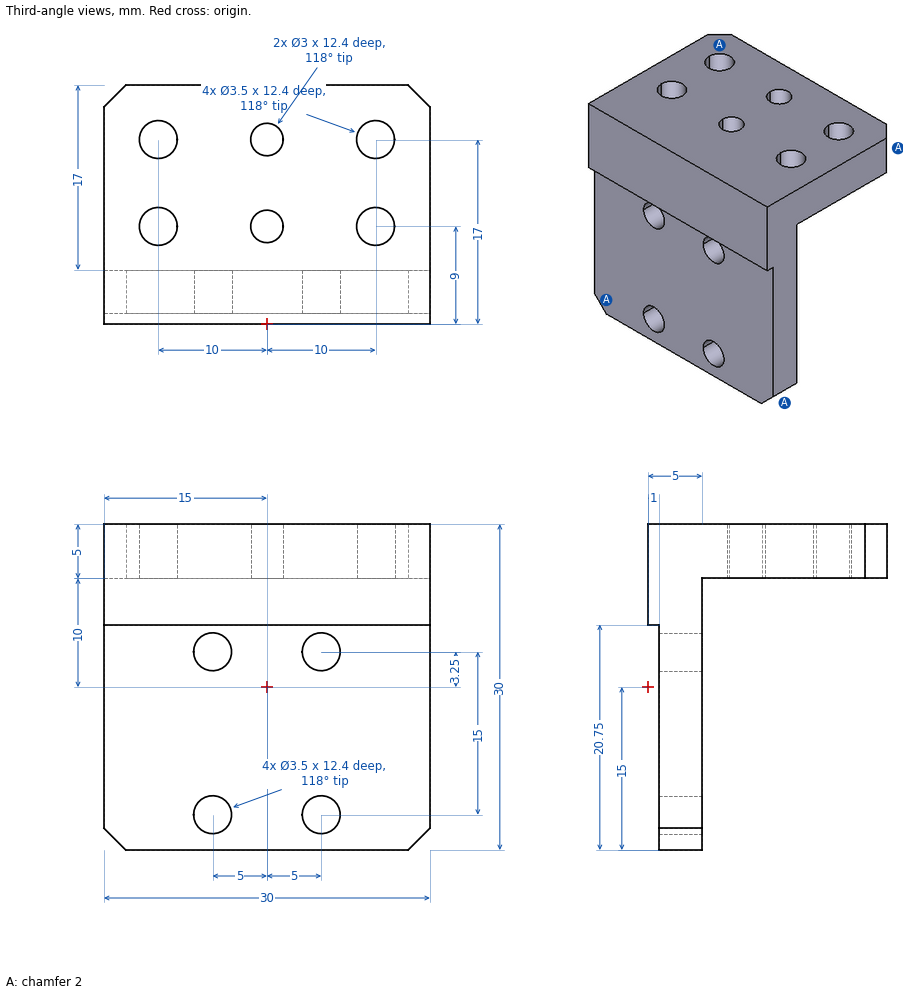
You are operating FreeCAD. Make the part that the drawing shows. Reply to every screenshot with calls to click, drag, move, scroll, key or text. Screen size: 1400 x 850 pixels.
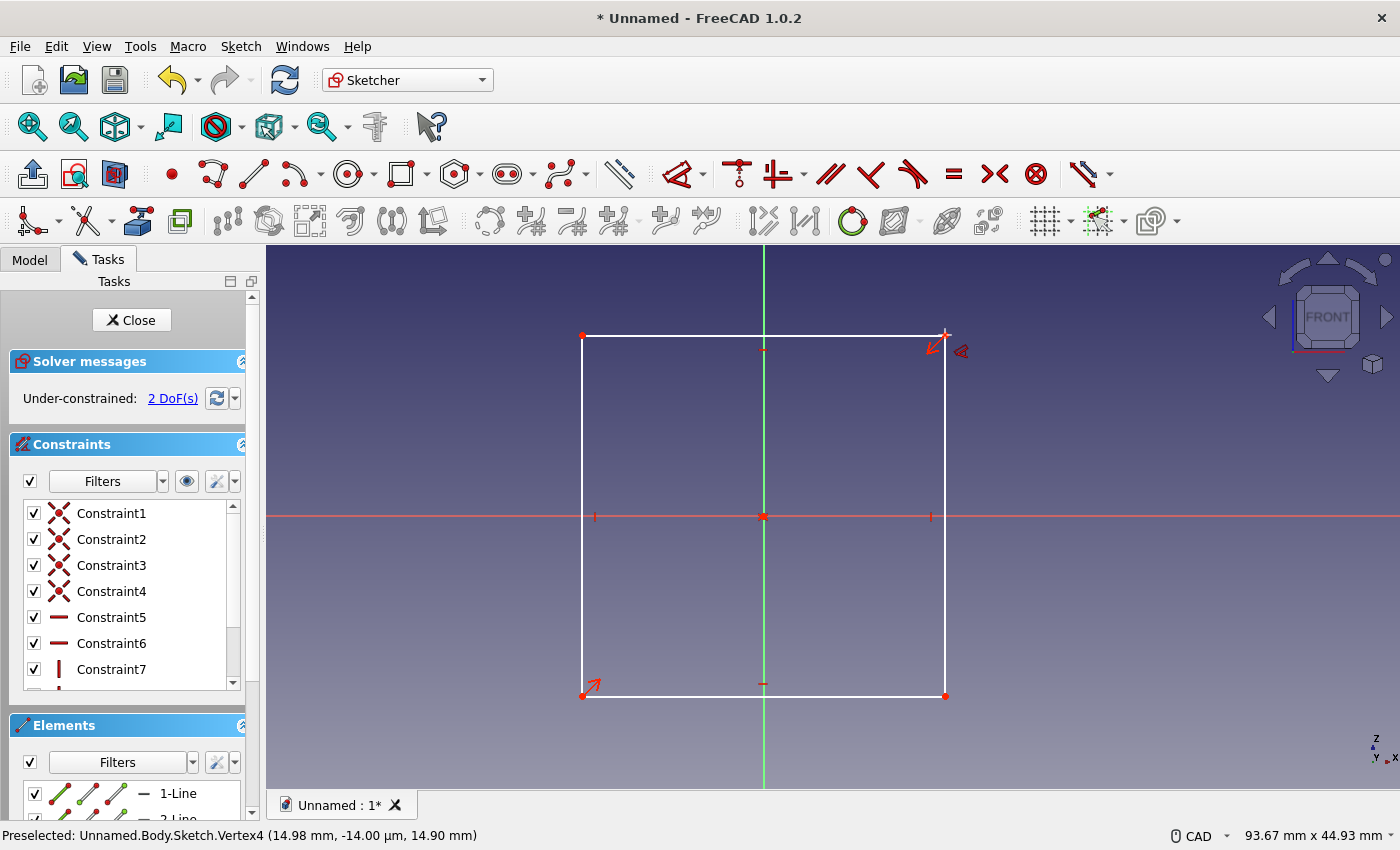
click(691, 697)
click(680, 731)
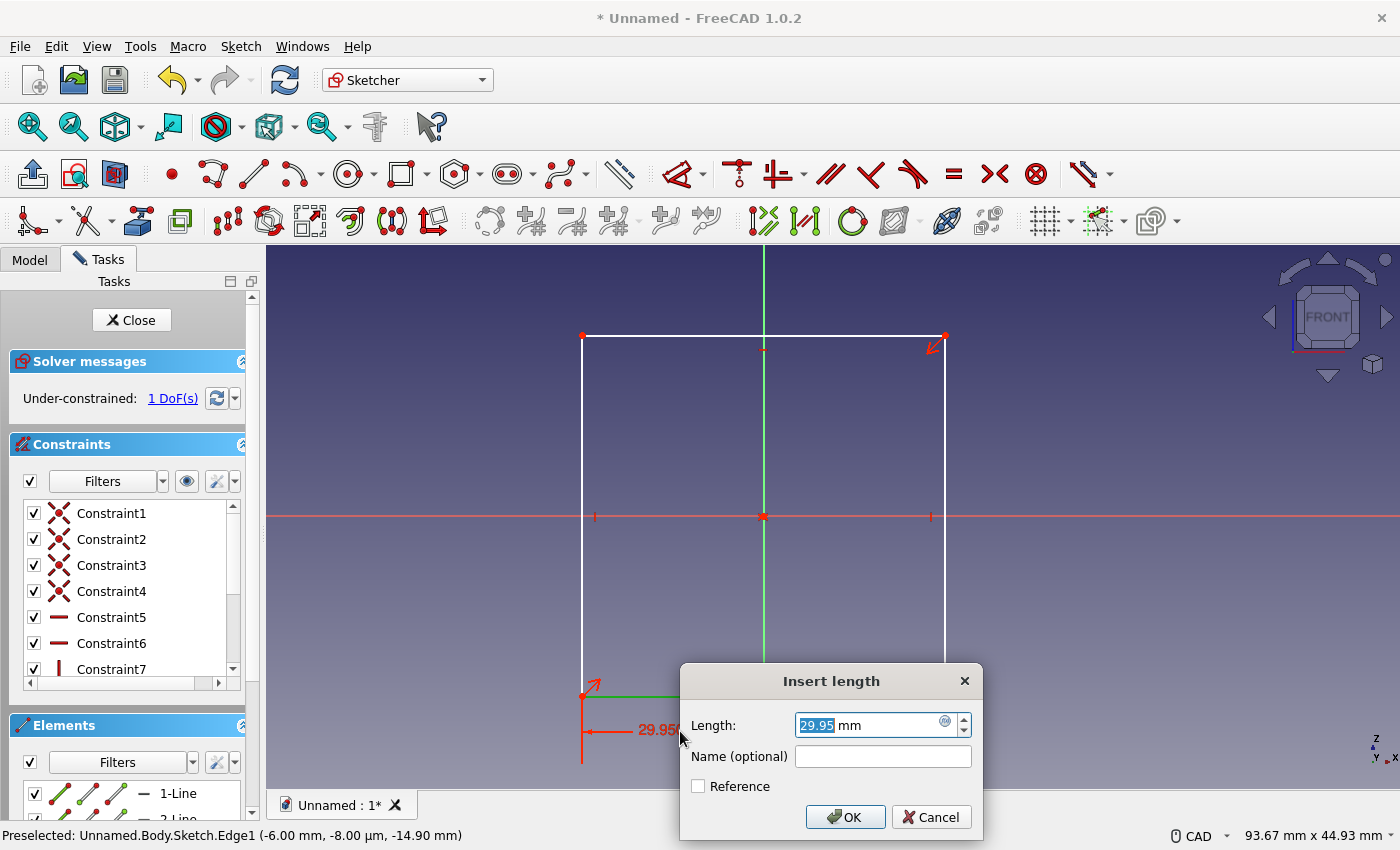
text(30)
key(Return)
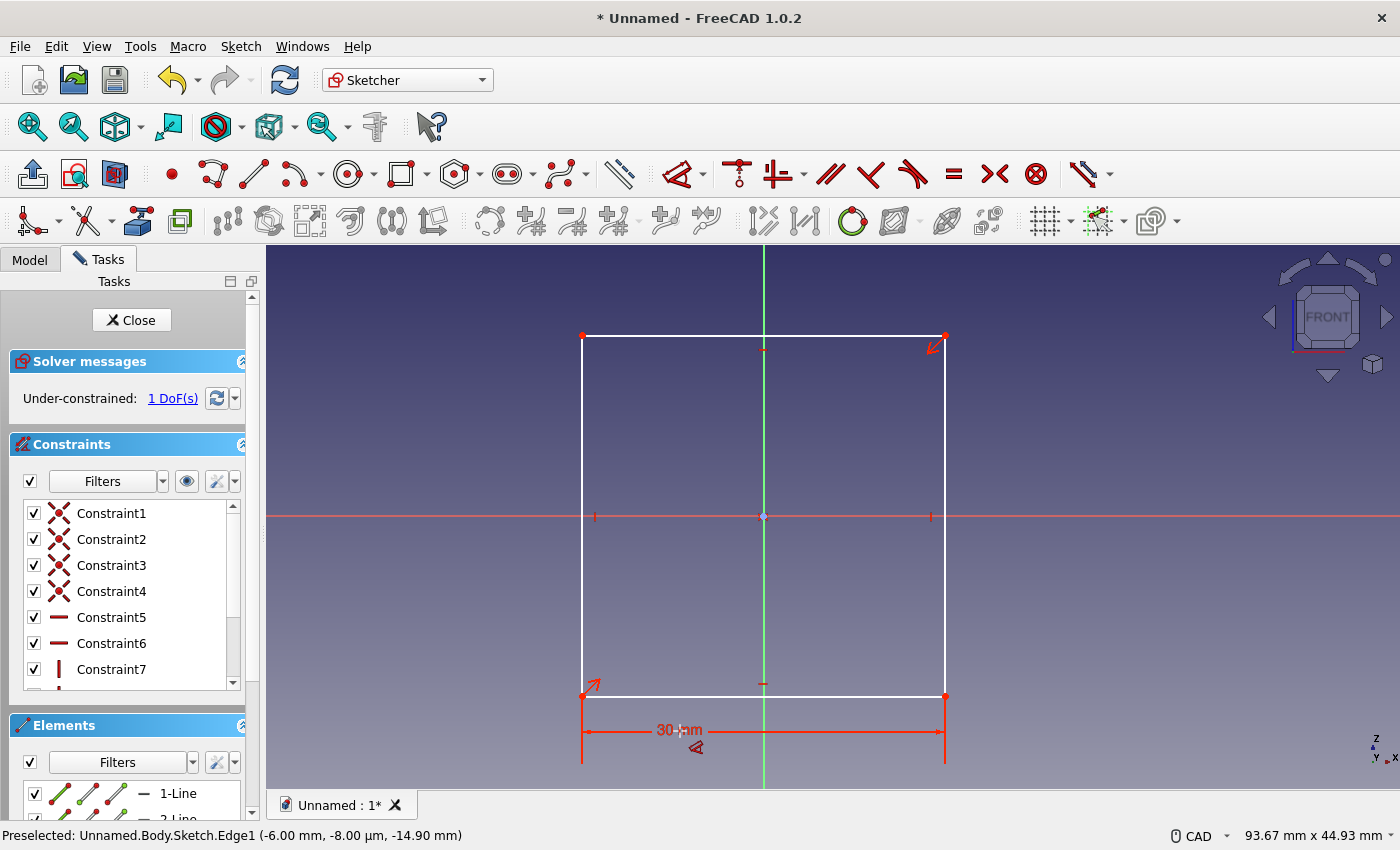
click(945, 589)
click(979, 433)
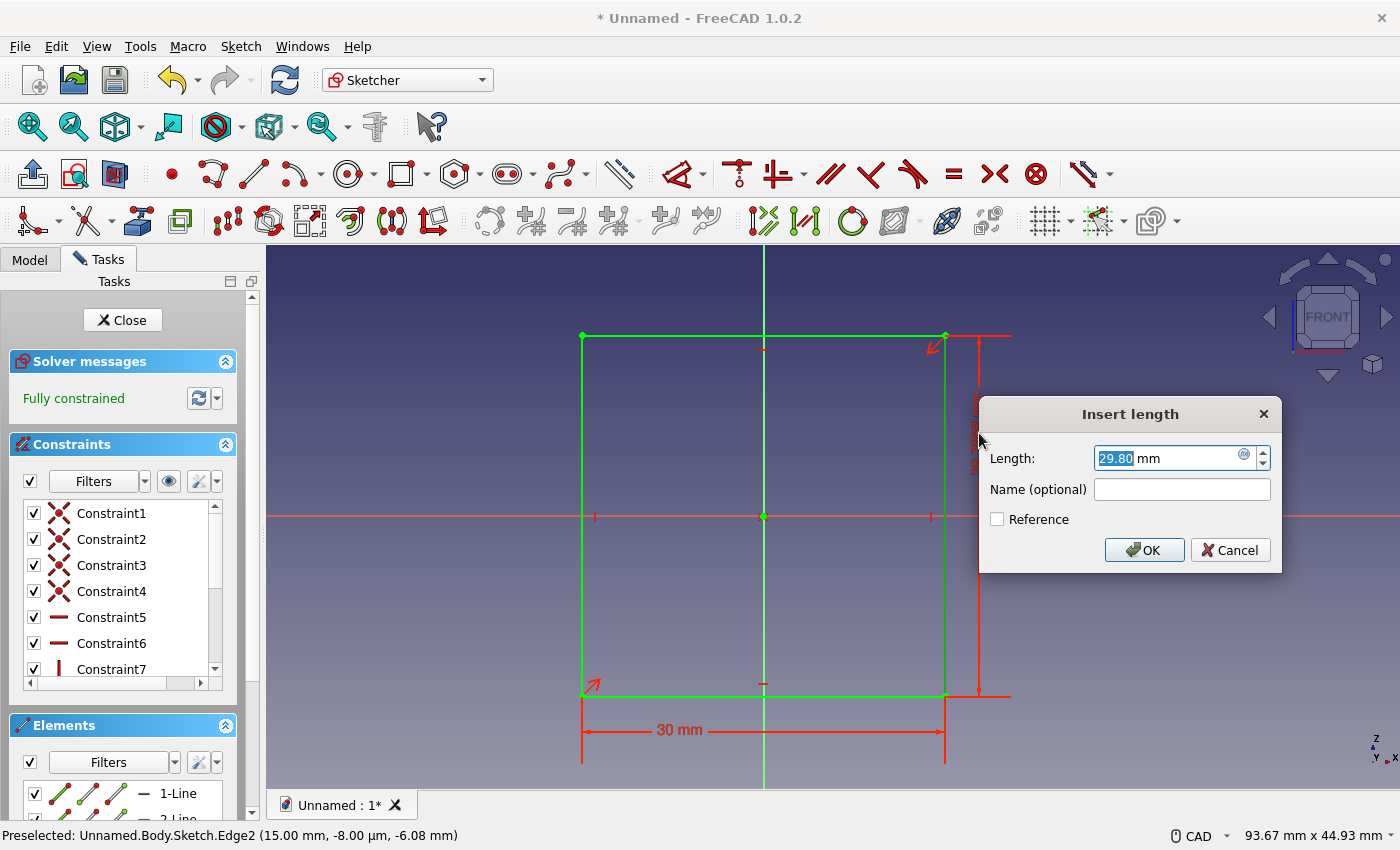
text(30)
key(Return)
key(Escape)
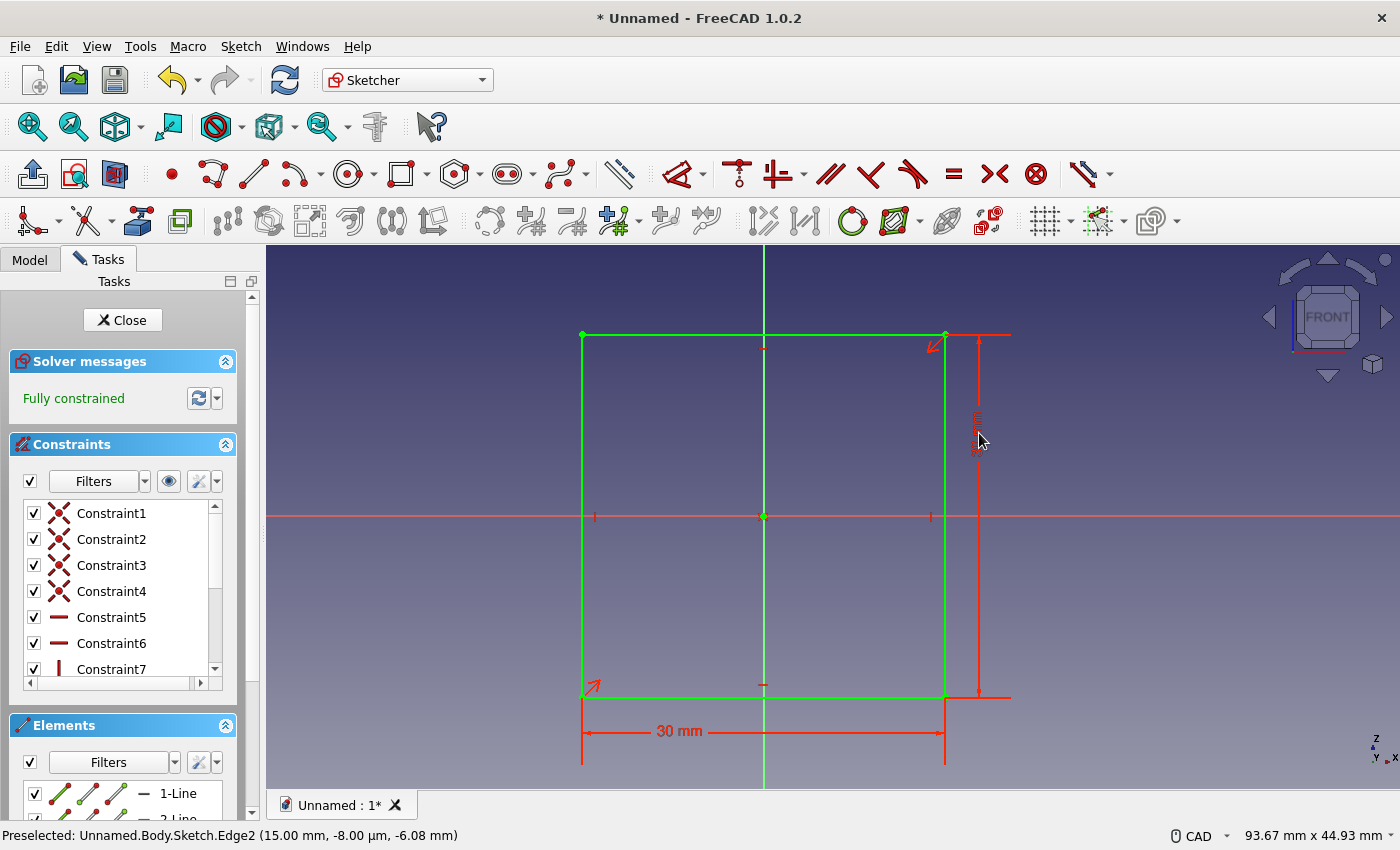
click(123, 320)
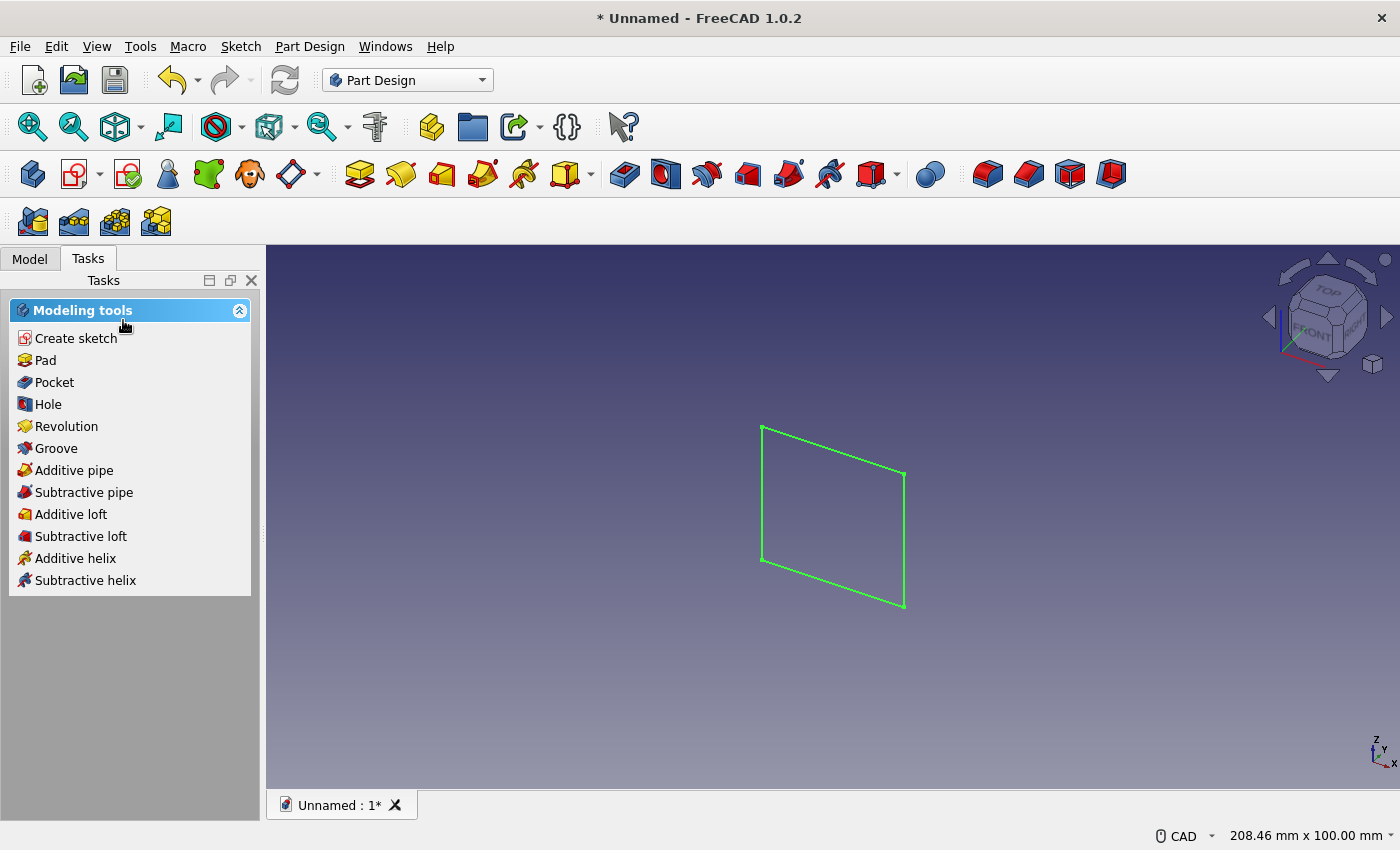
click(360, 174)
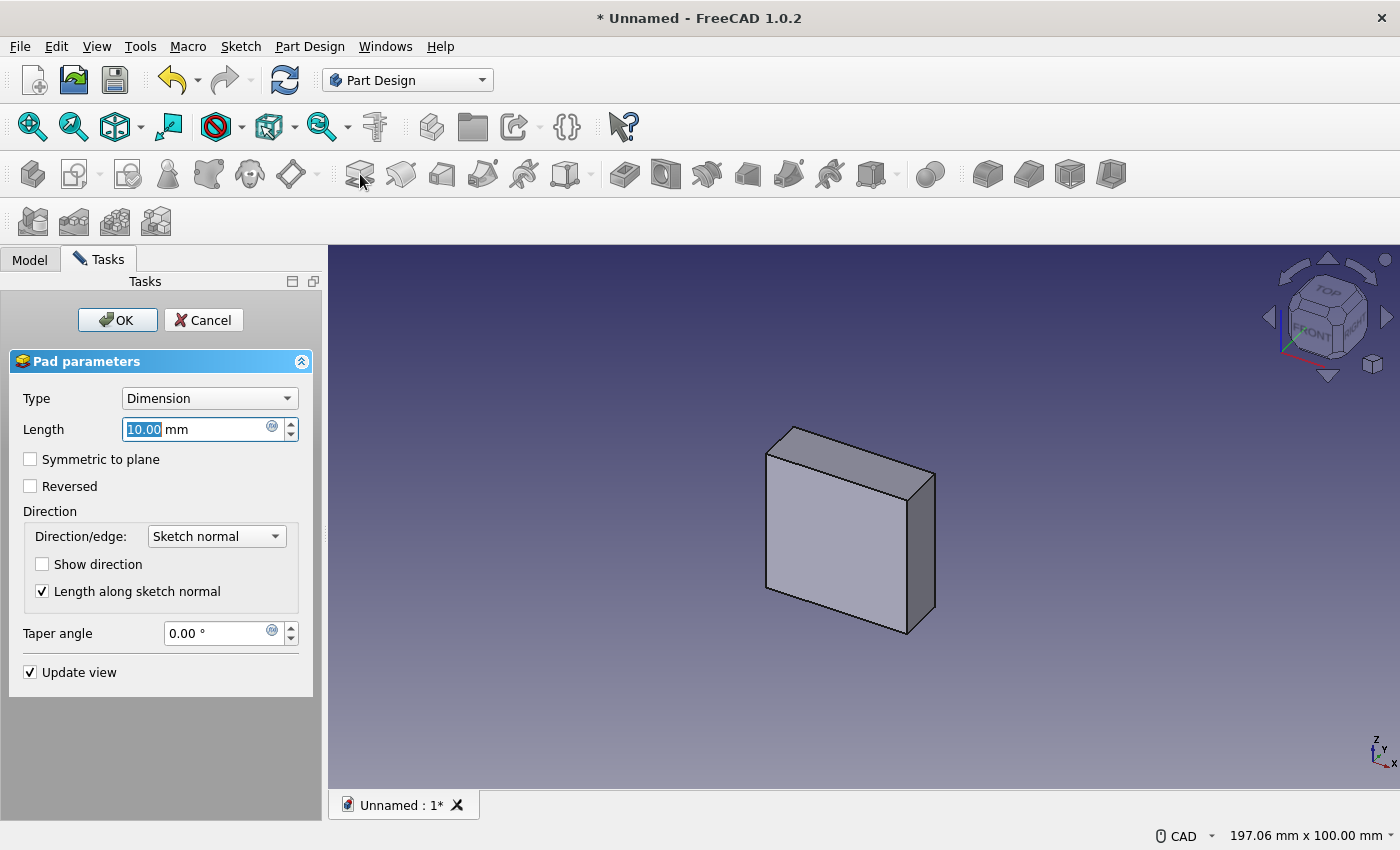
text(5)
key(Tab)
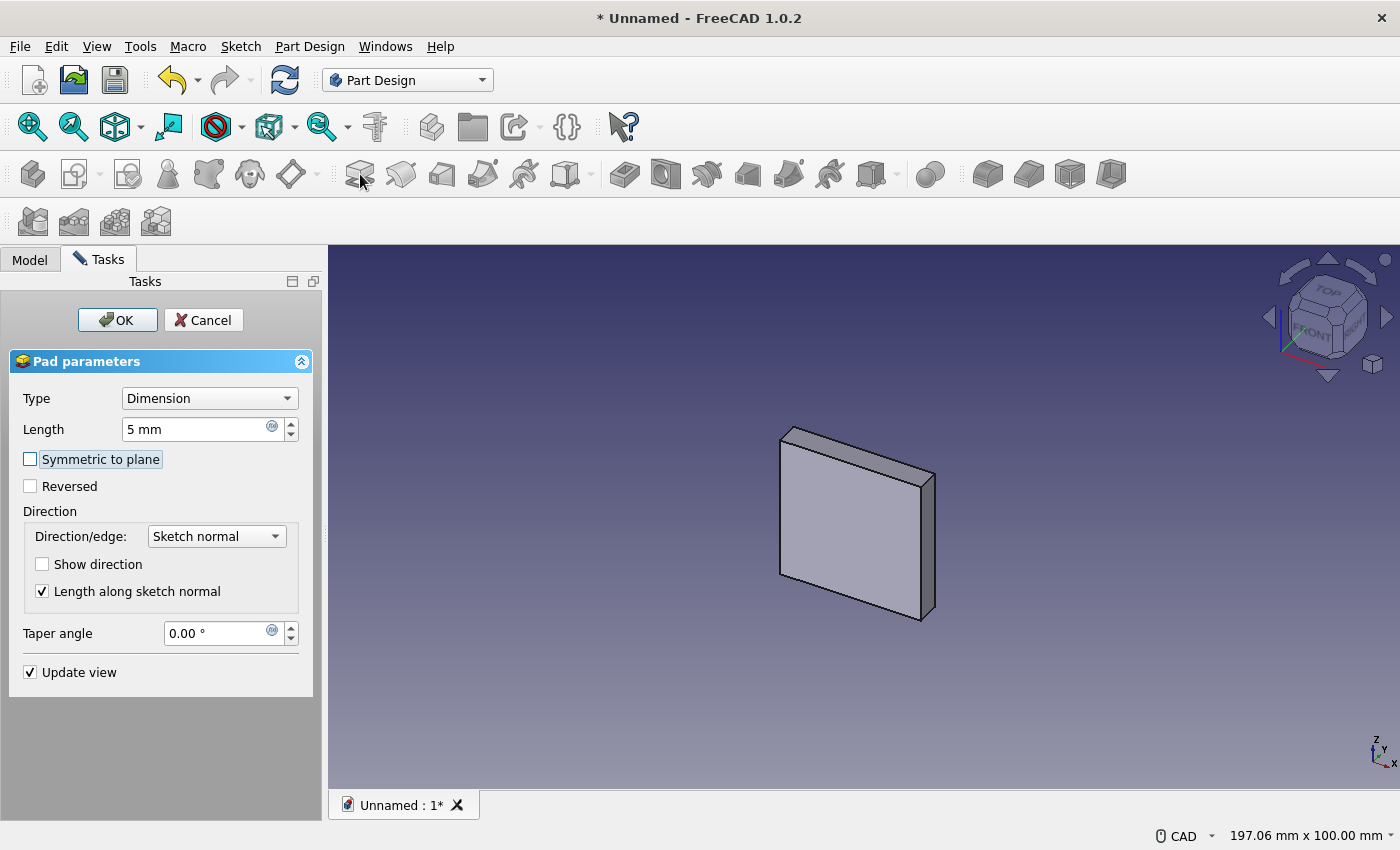
click(31, 486)